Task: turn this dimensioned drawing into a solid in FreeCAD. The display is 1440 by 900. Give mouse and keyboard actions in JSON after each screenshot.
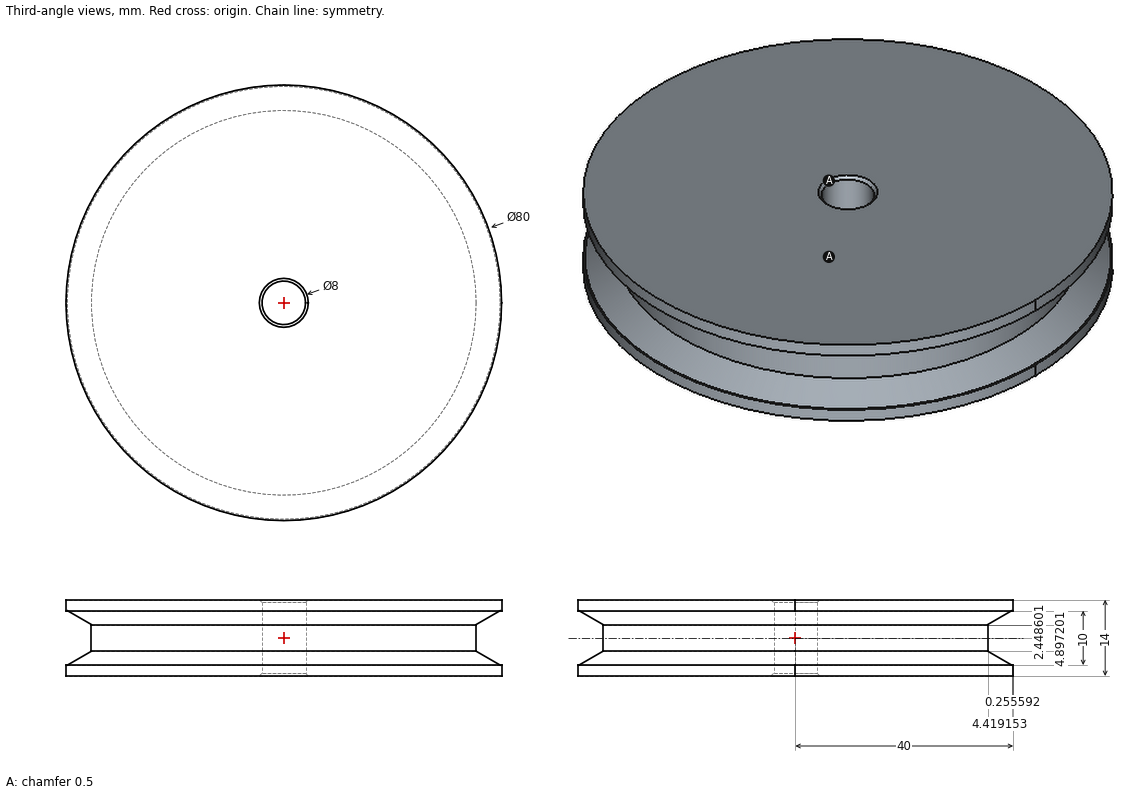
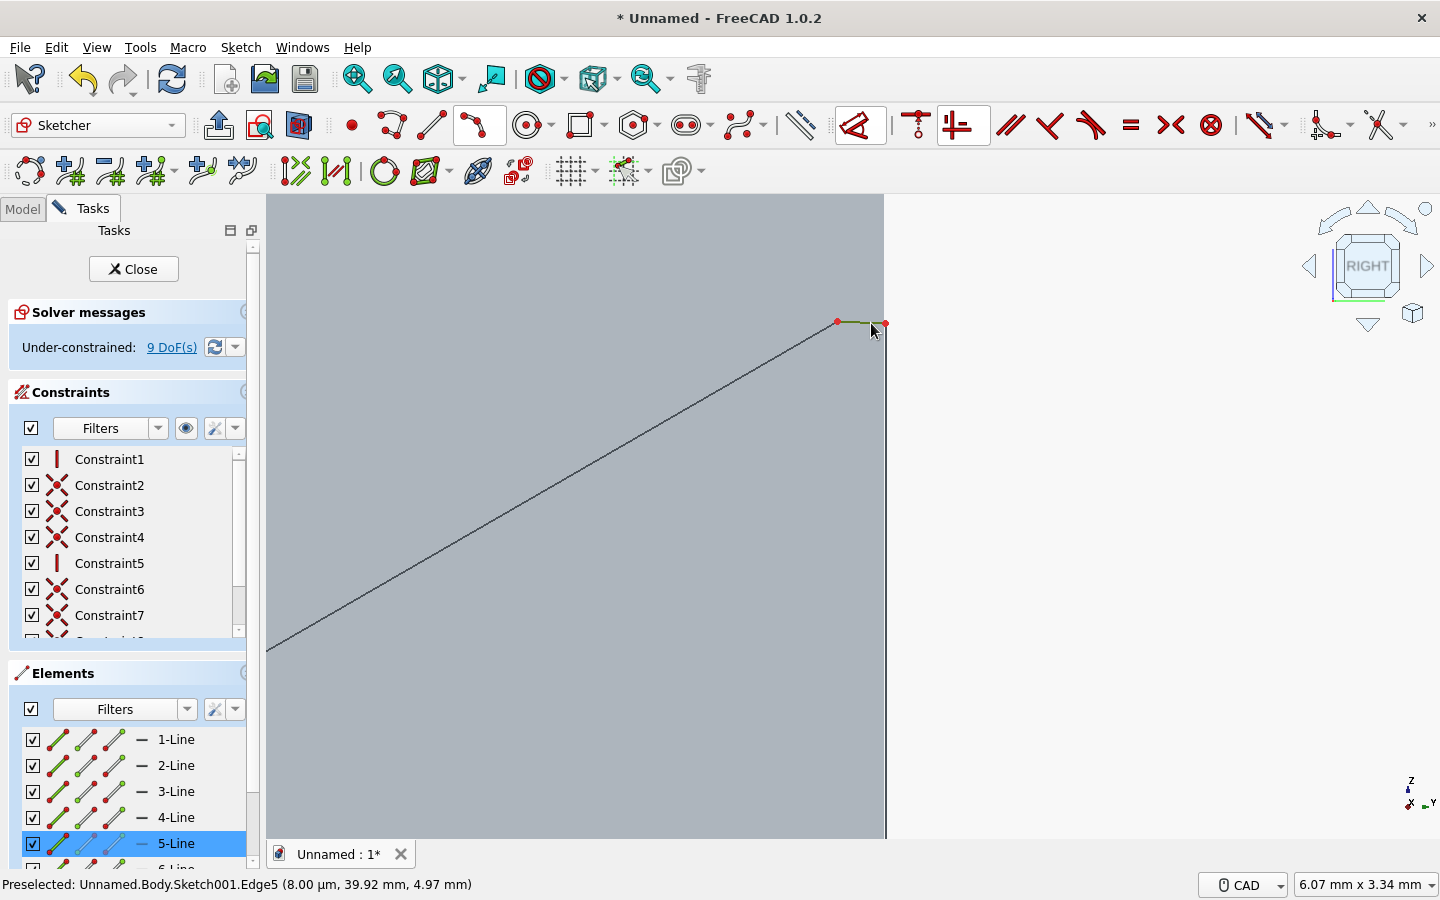
{"action": "key", "text": "h"}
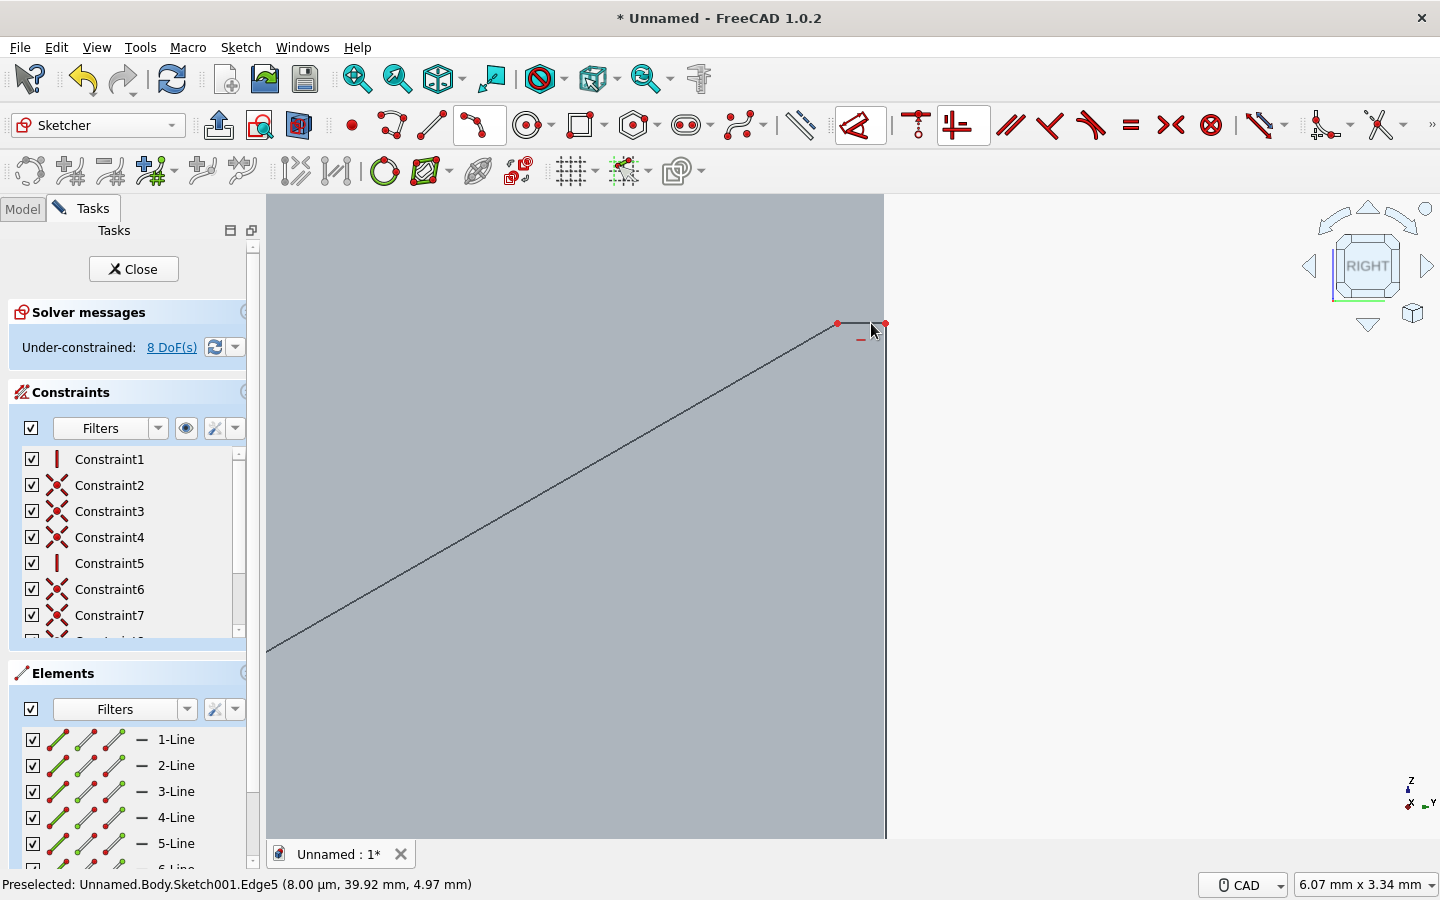
{"action": "scroll", "coordinate": [873, 322], "scroll_direction": "down", "scroll_amount": 8}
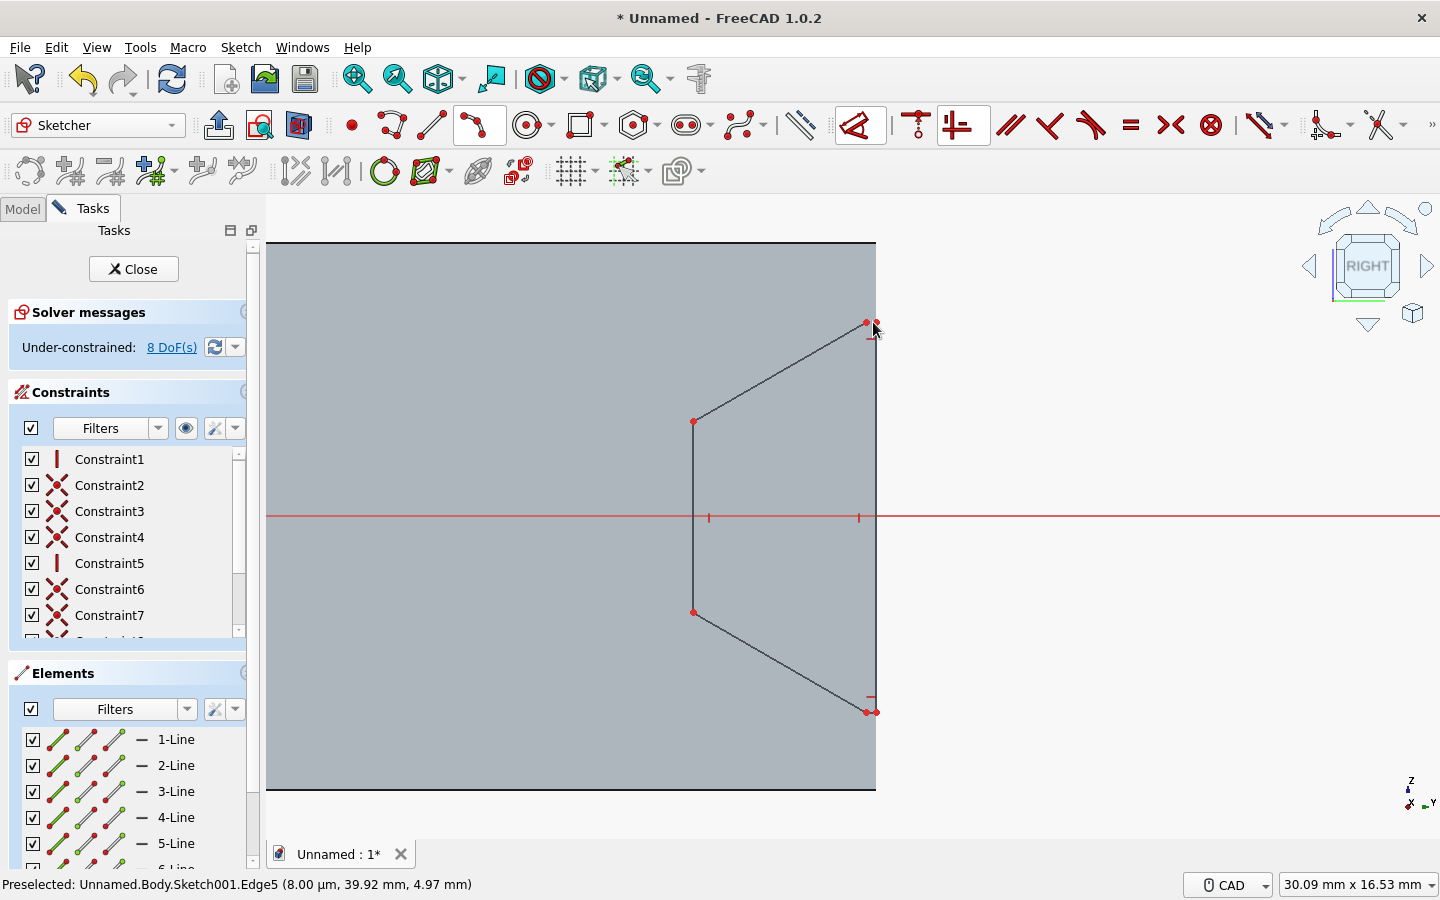
{"action": "scroll", "coordinate": [866, 713], "scroll_direction": "up", "scroll_amount": 2}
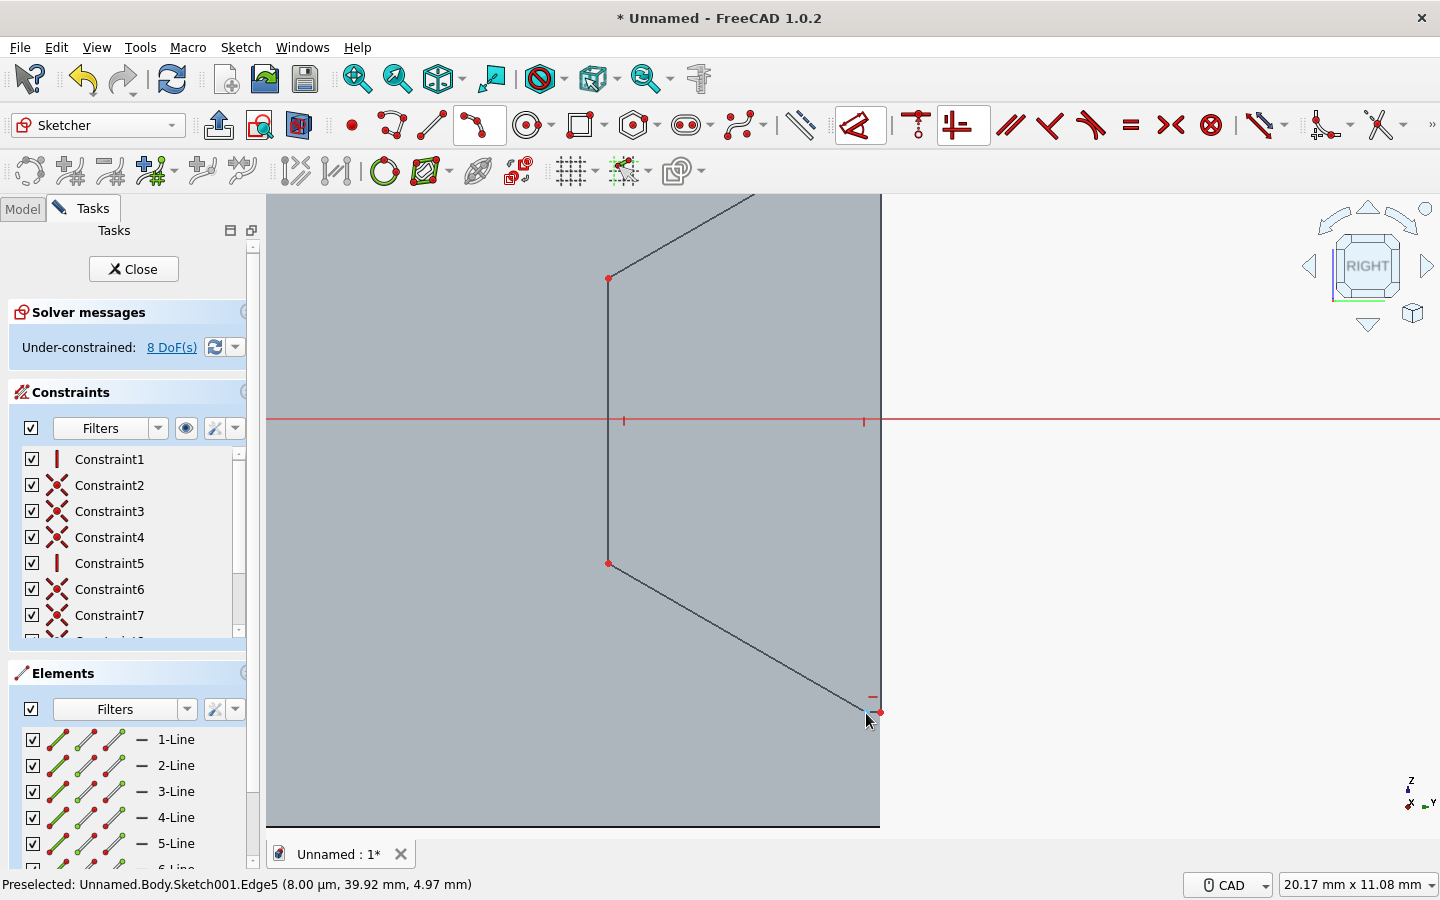
{"action": "left_click", "coordinate": [866, 712]}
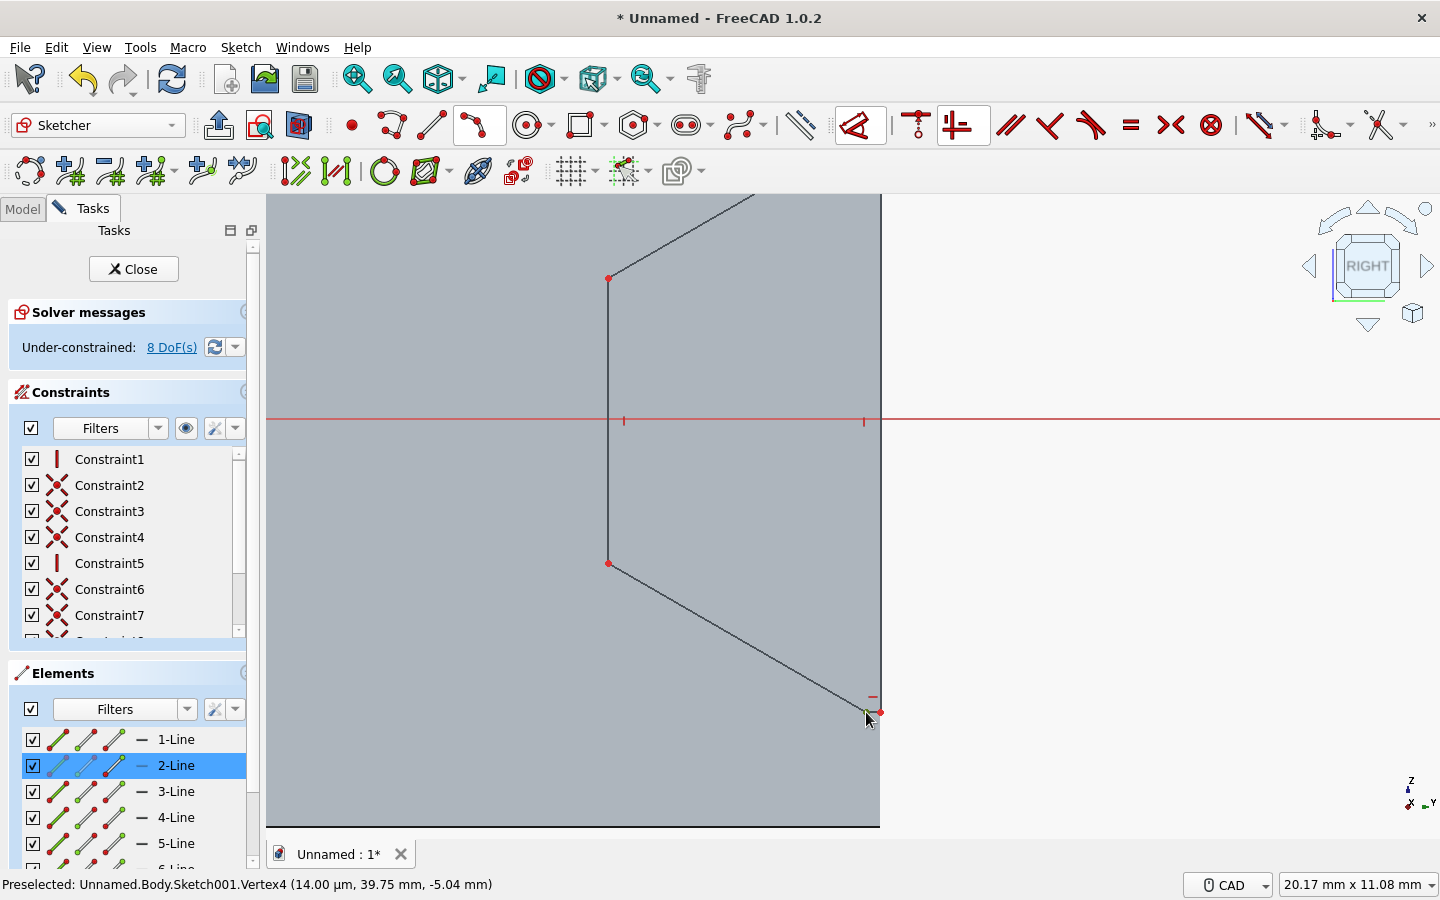
{"action": "scroll", "coordinate": [865, 714], "scroll_direction": "down", "scroll_amount": 2}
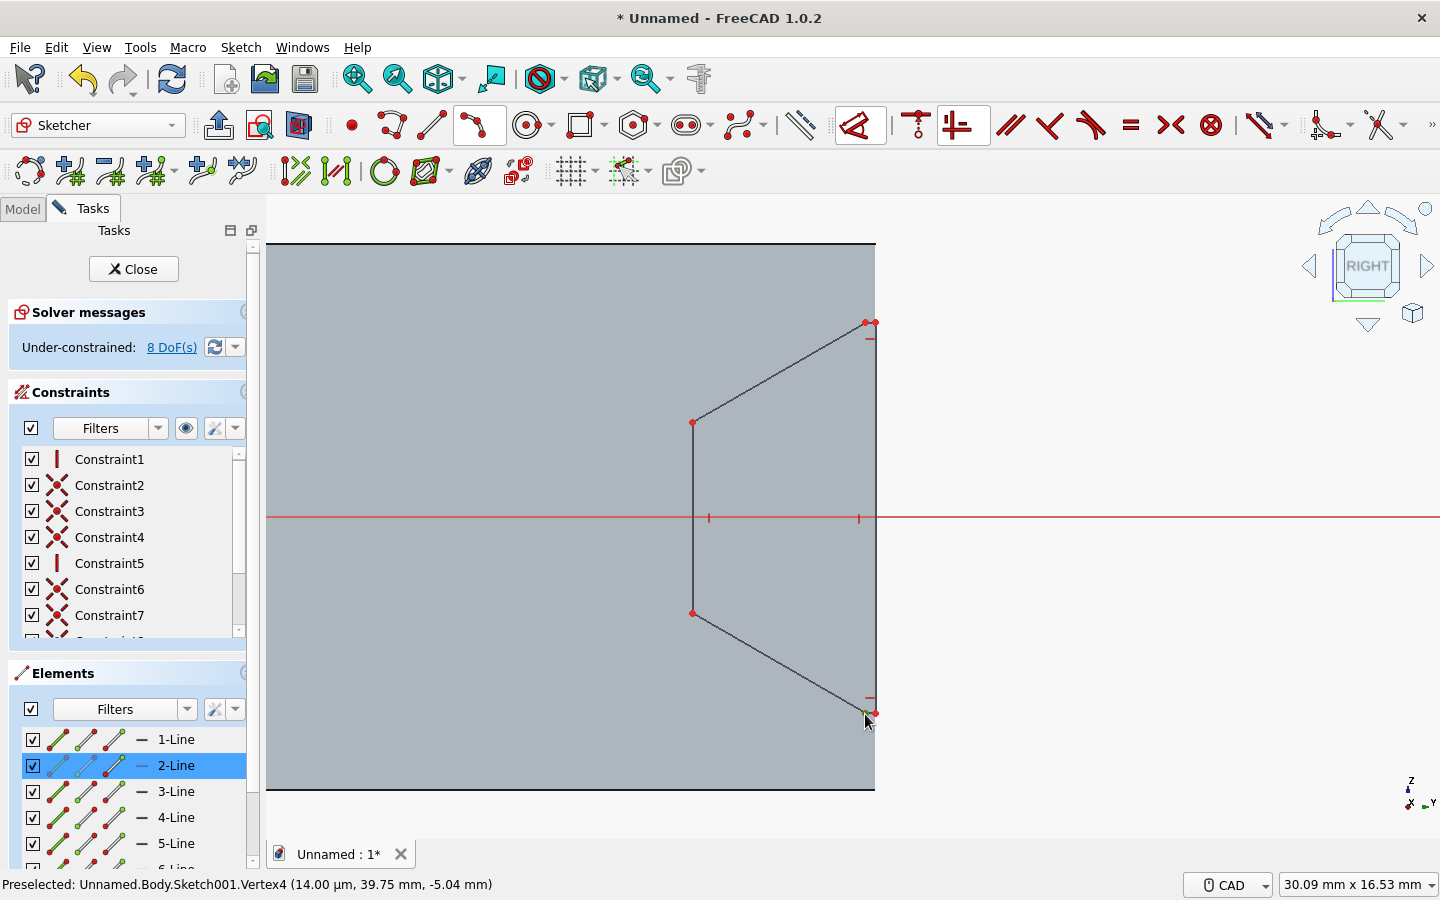
{"action": "scroll", "coordinate": [866, 323], "scroll_direction": "up", "scroll_amount": 2}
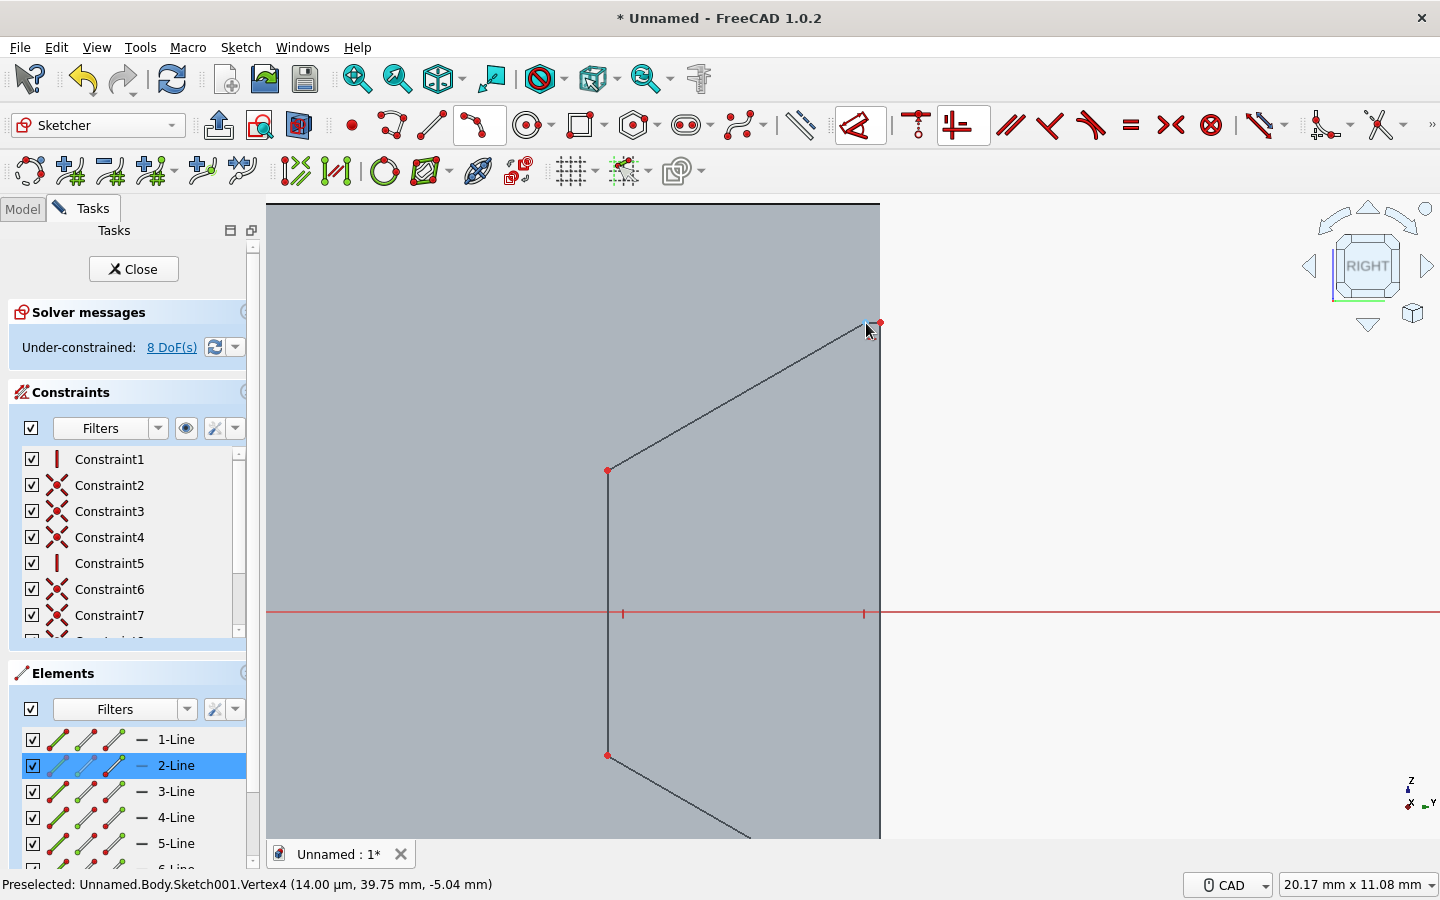
{"action": "left_click", "coordinate": [866, 323]}